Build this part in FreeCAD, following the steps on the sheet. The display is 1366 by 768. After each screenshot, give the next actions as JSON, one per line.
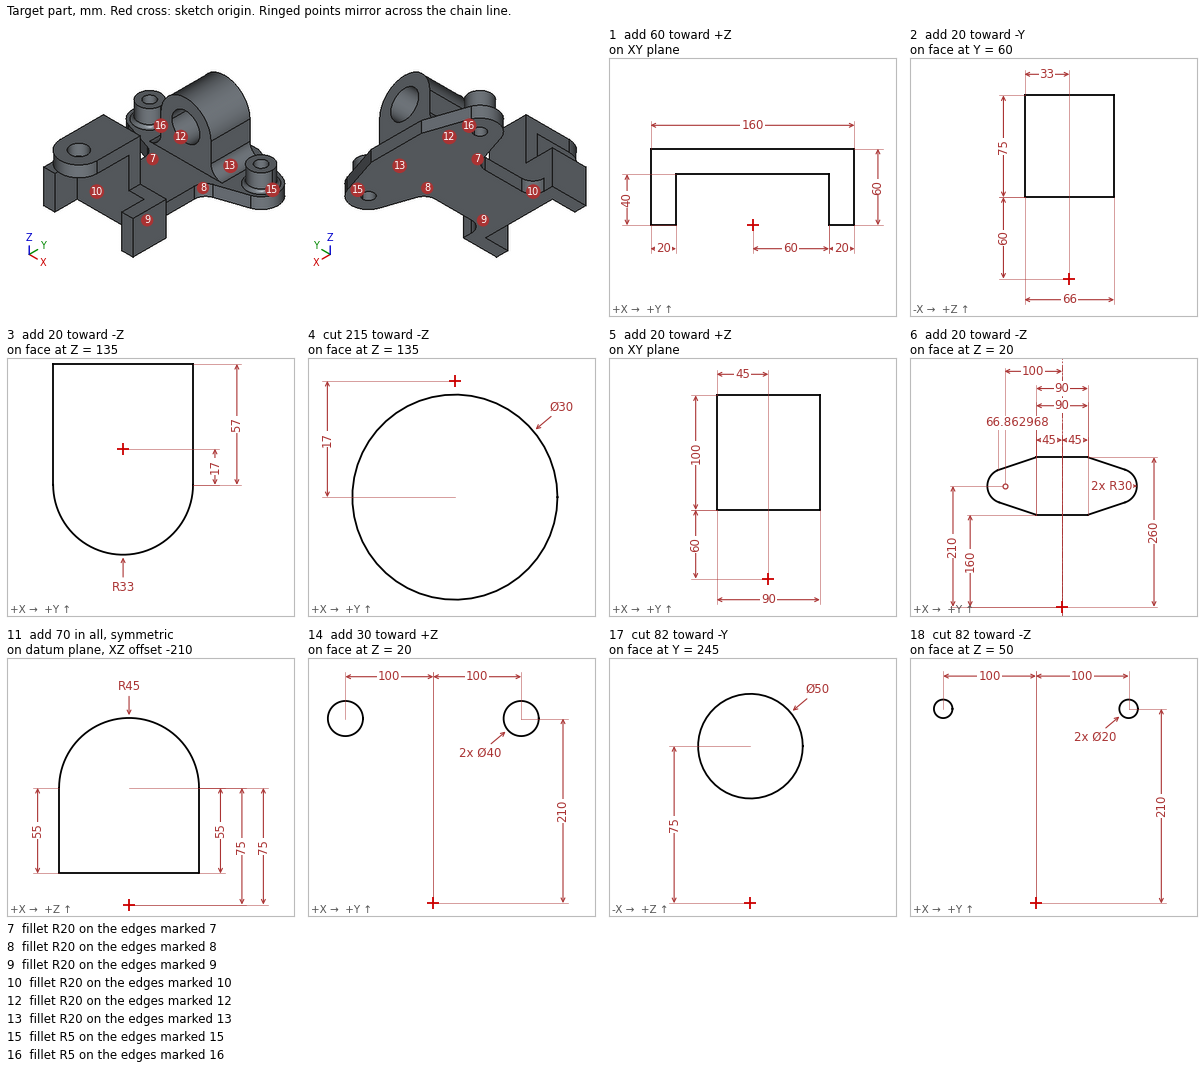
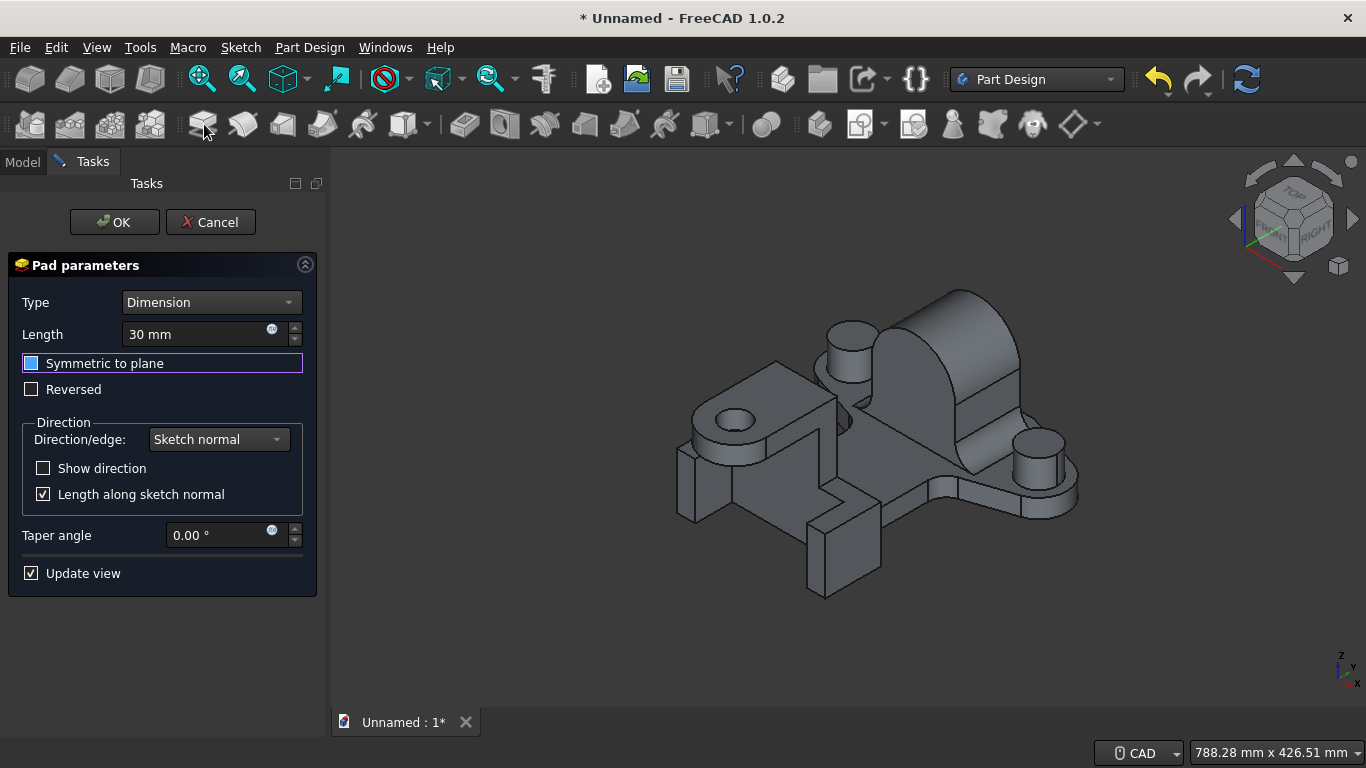
{"action": "left_click", "coordinate": [115, 222]}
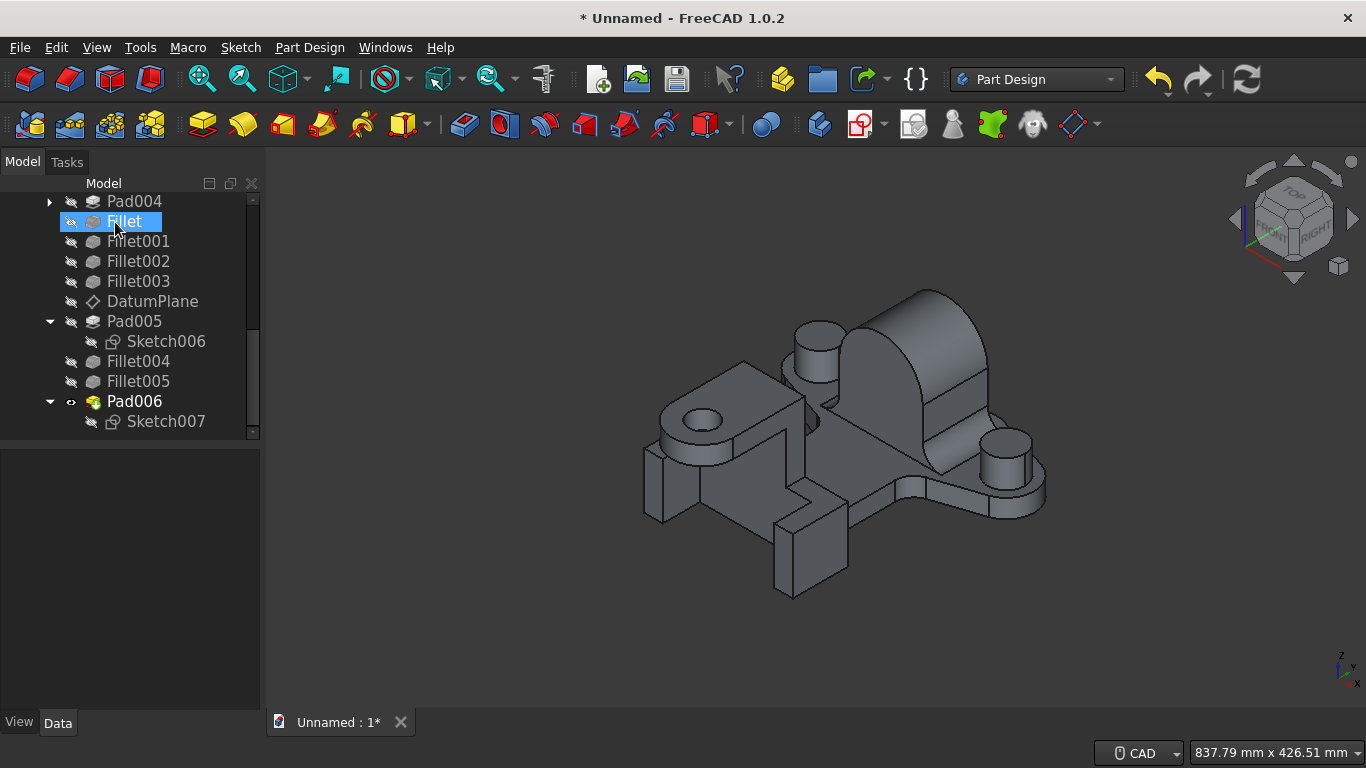
{"action": "left_click", "coordinate": [983, 481]}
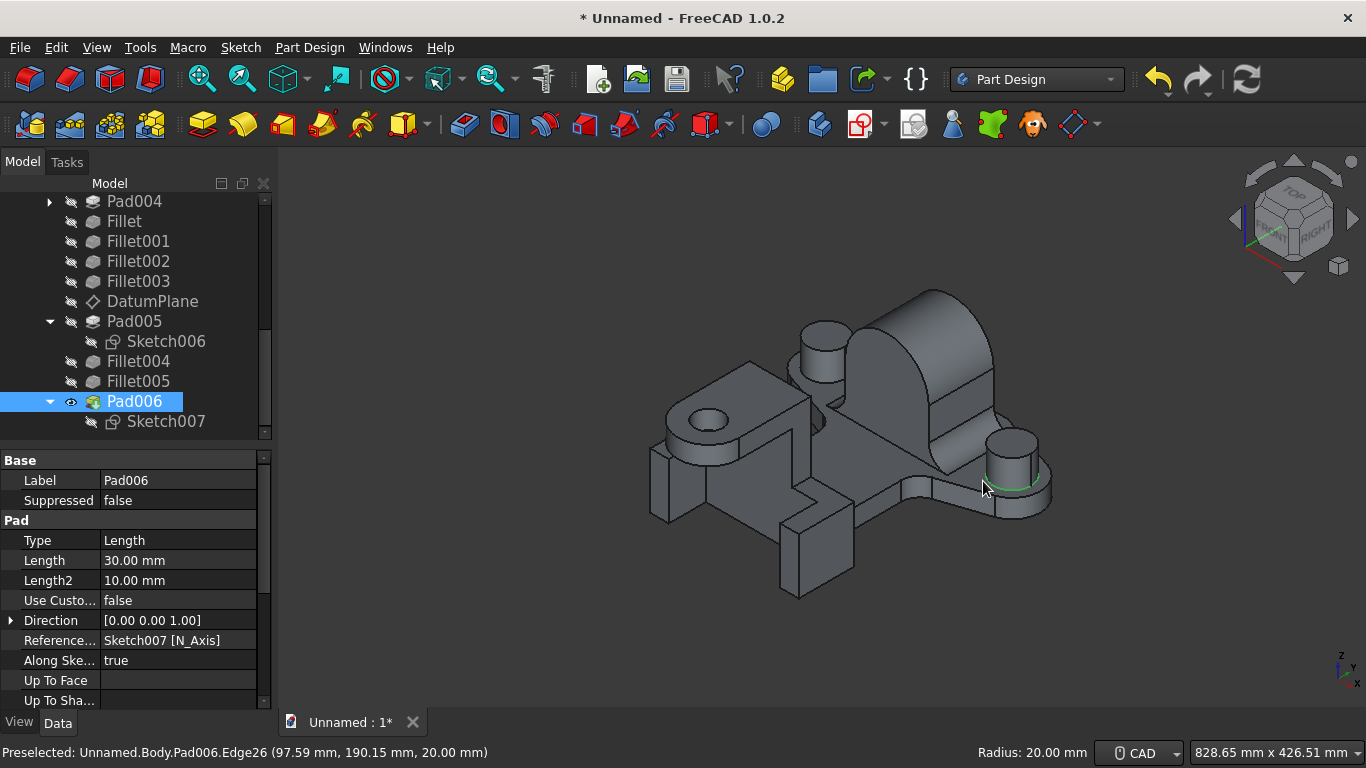
{"action": "left_click", "coordinate": [30, 80]}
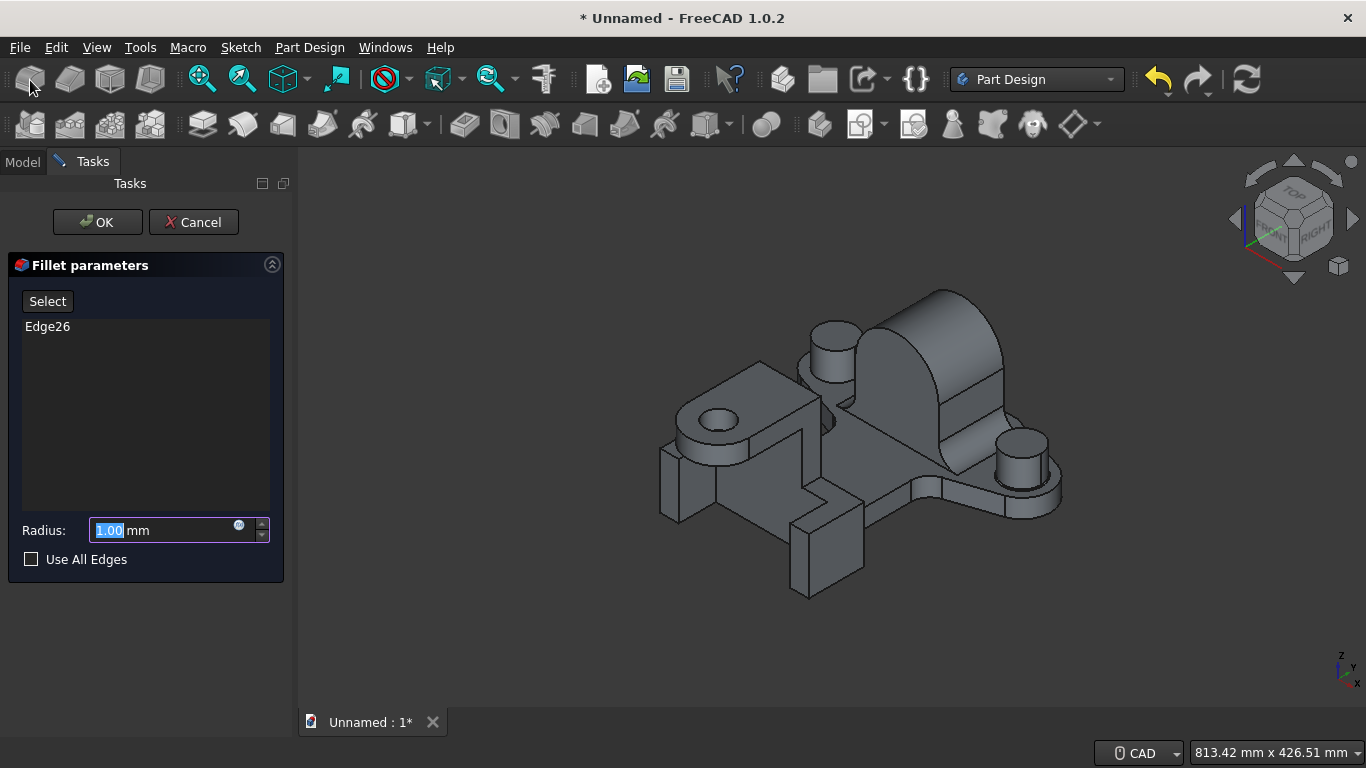
{"action": "type", "text": "5"}
{"action": "key", "text": "Tab"}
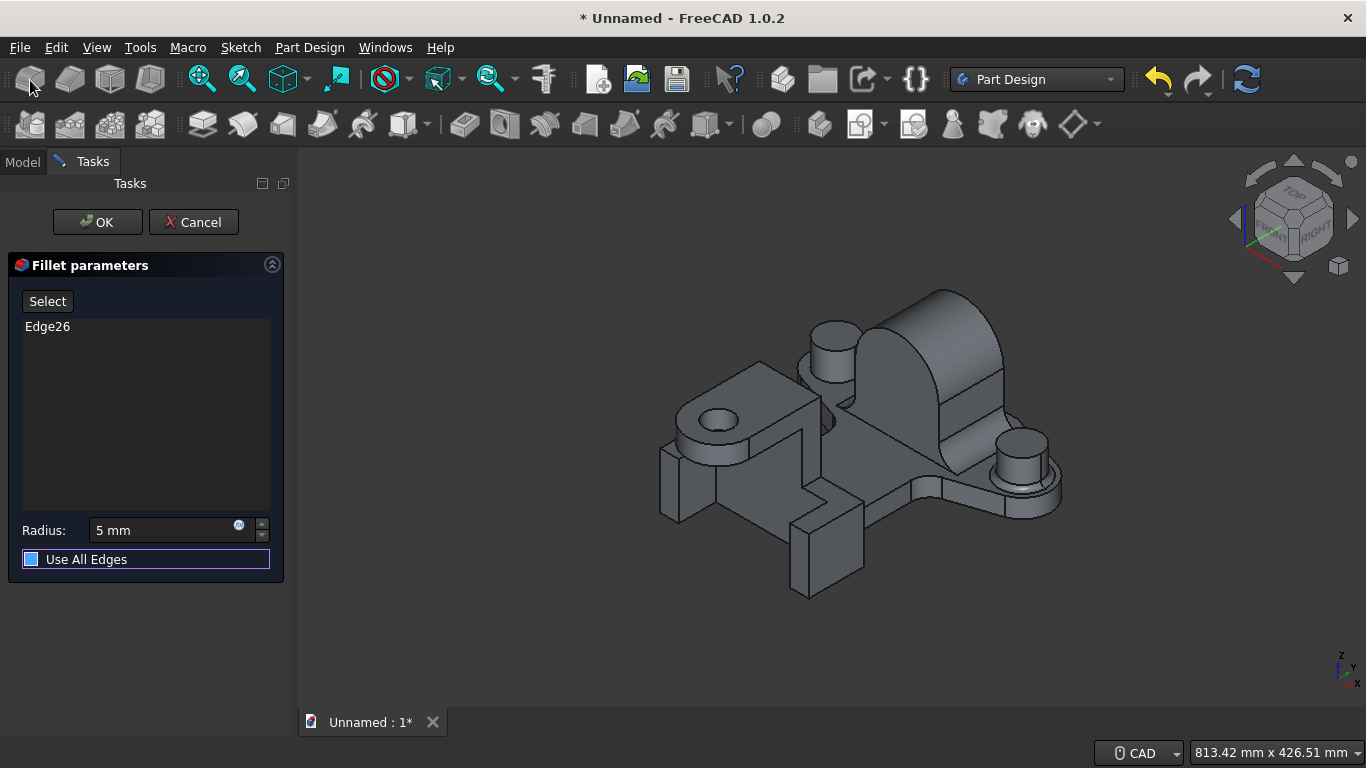
{"action": "left_click", "coordinate": [98, 222]}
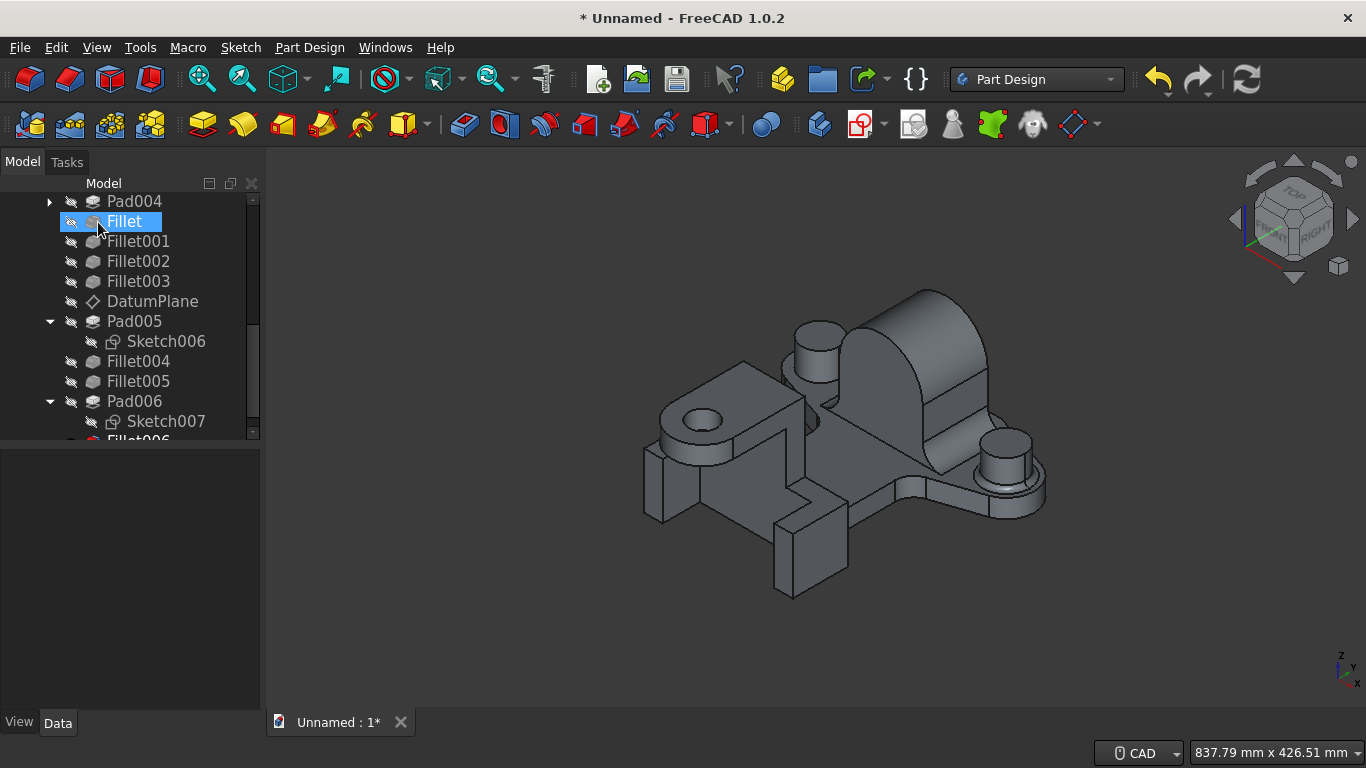
{"action": "key", "text": "2"}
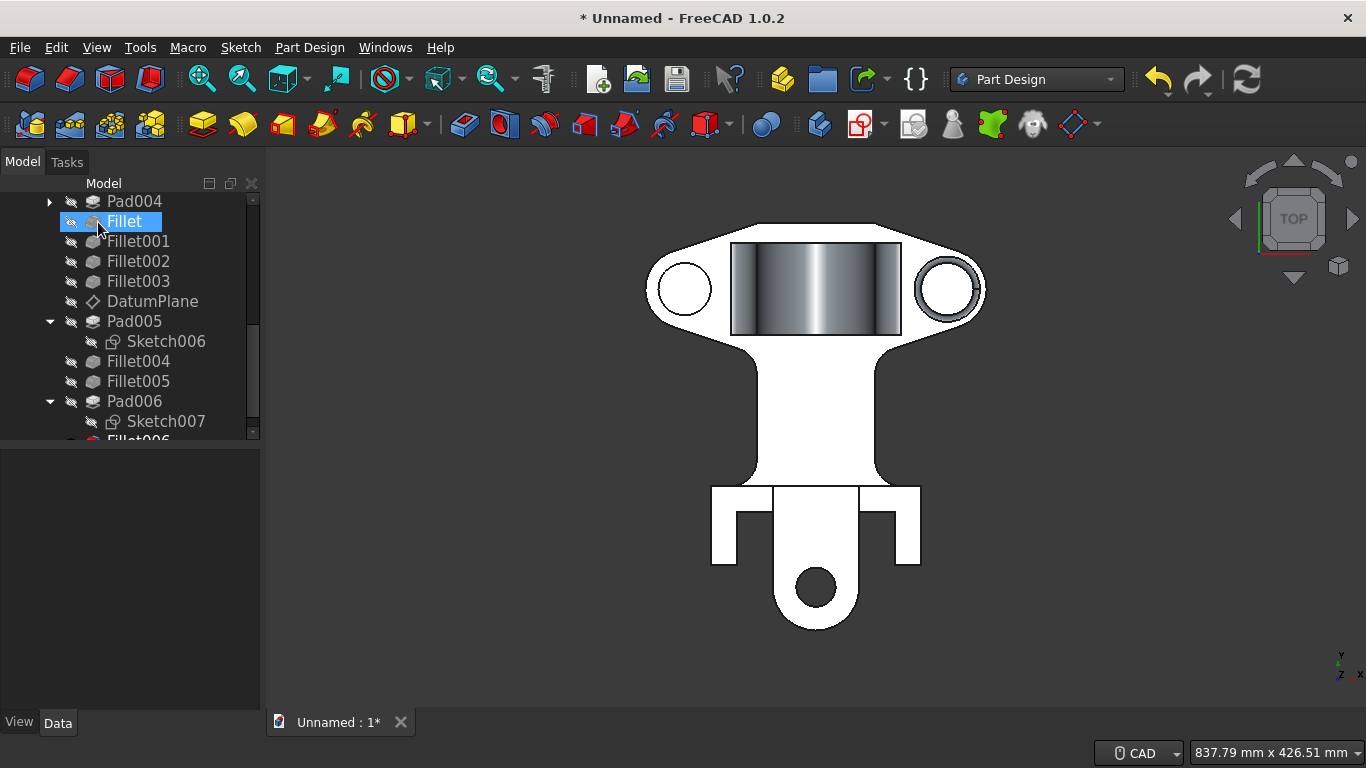
{"action": "key", "text": "0"}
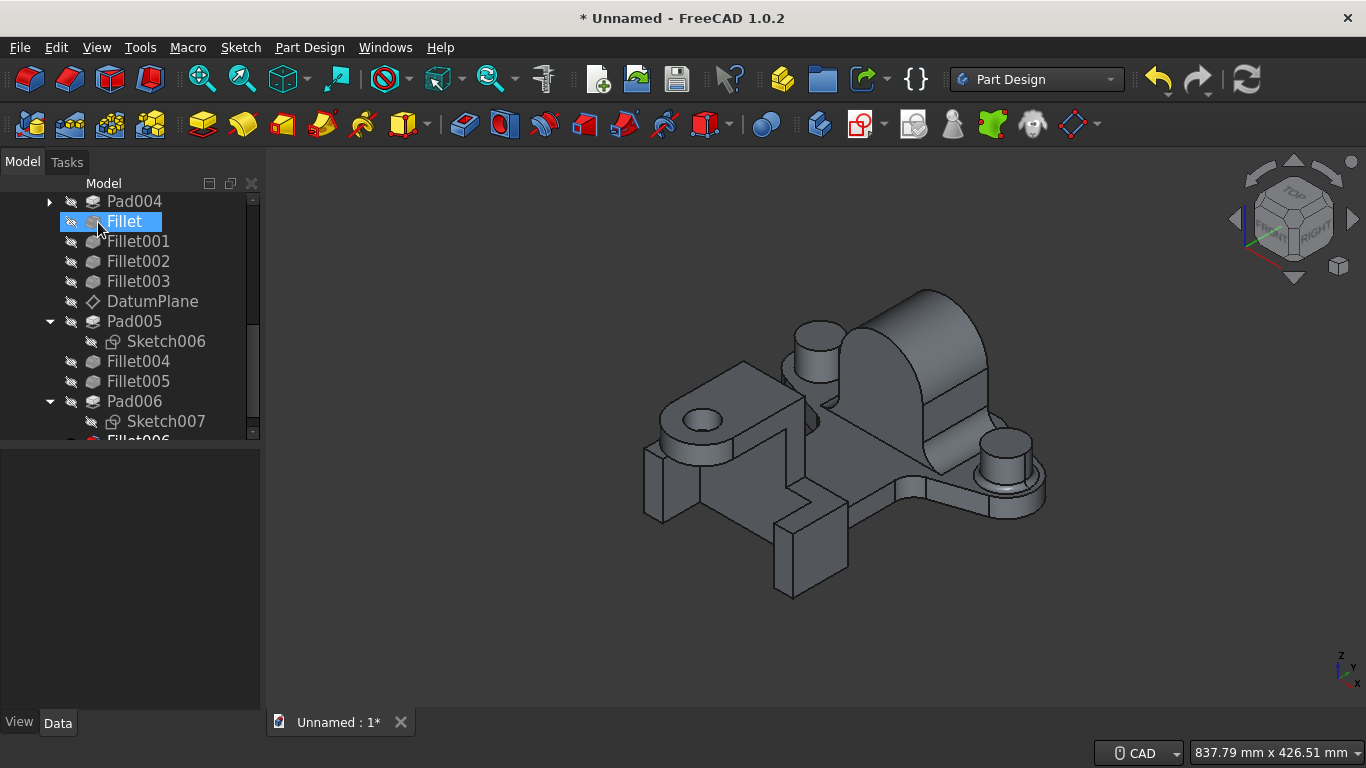
{"action": "key", "text": "1"}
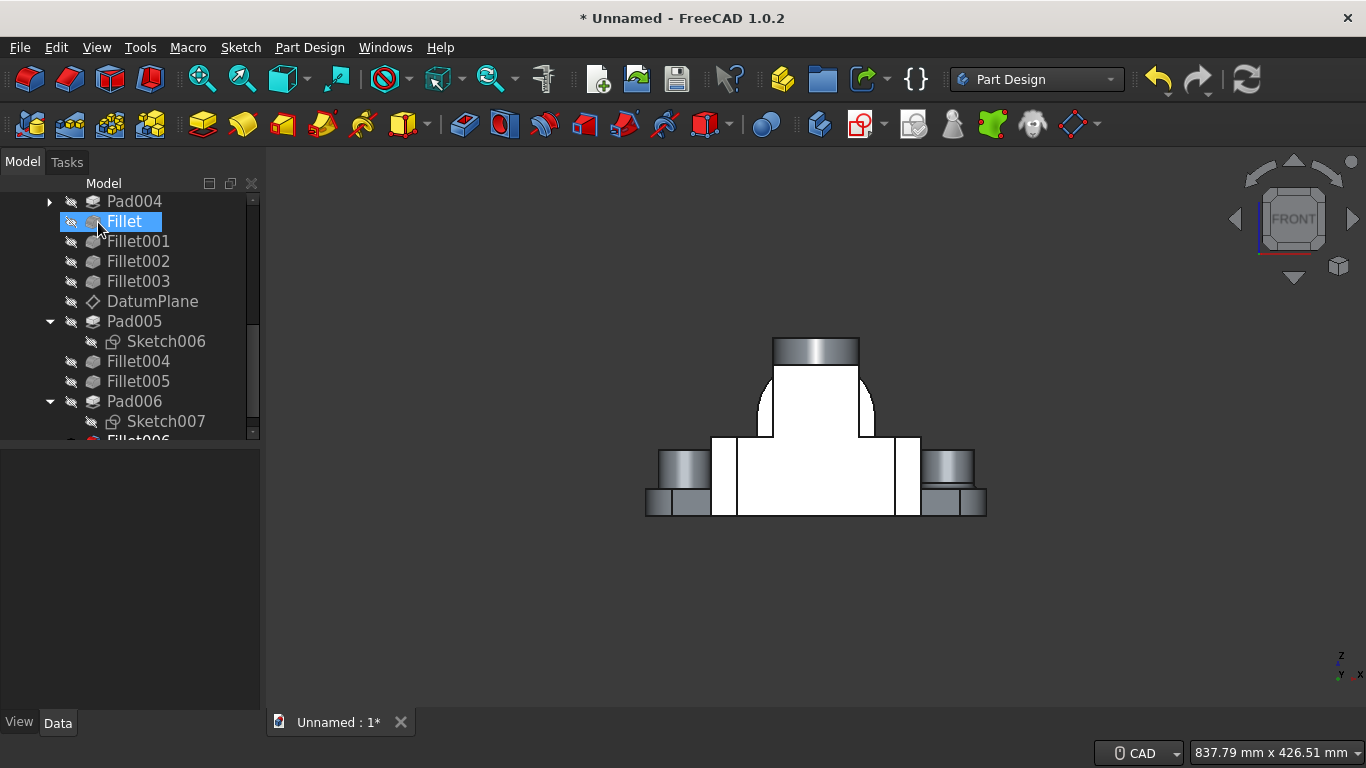
{"action": "left_click", "coordinate": [204, 80]}